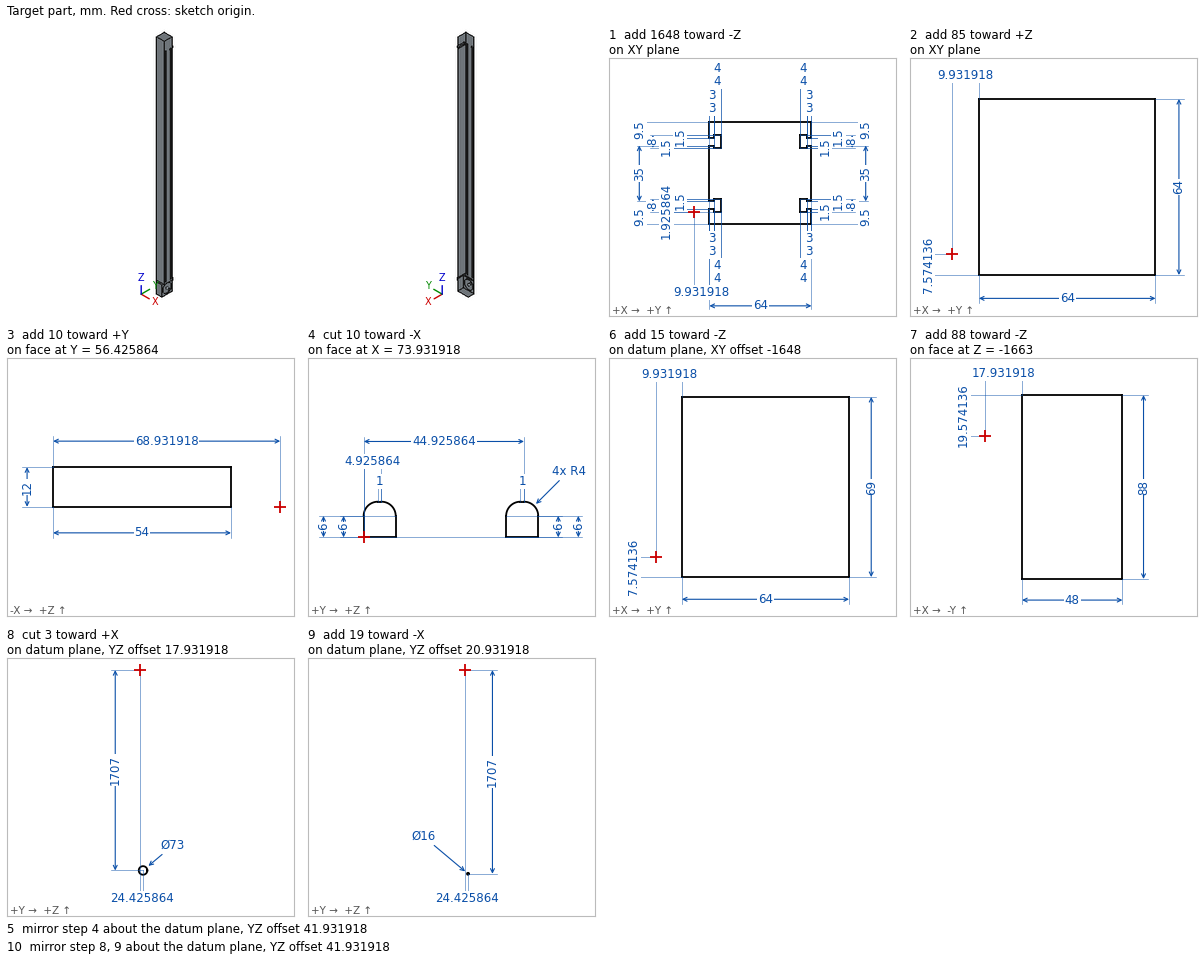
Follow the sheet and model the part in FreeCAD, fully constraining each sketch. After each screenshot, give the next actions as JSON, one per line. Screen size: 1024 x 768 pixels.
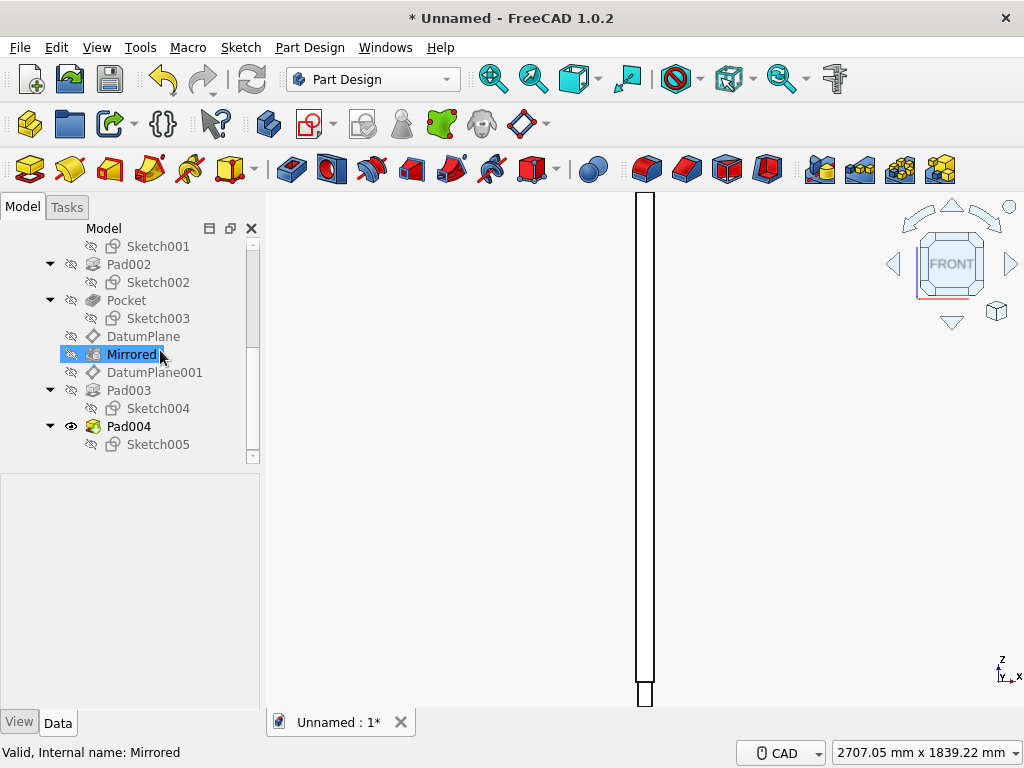
{"action": "scroll", "coordinate": [160, 350], "scroll_direction": "up", "scroll_amount": 15}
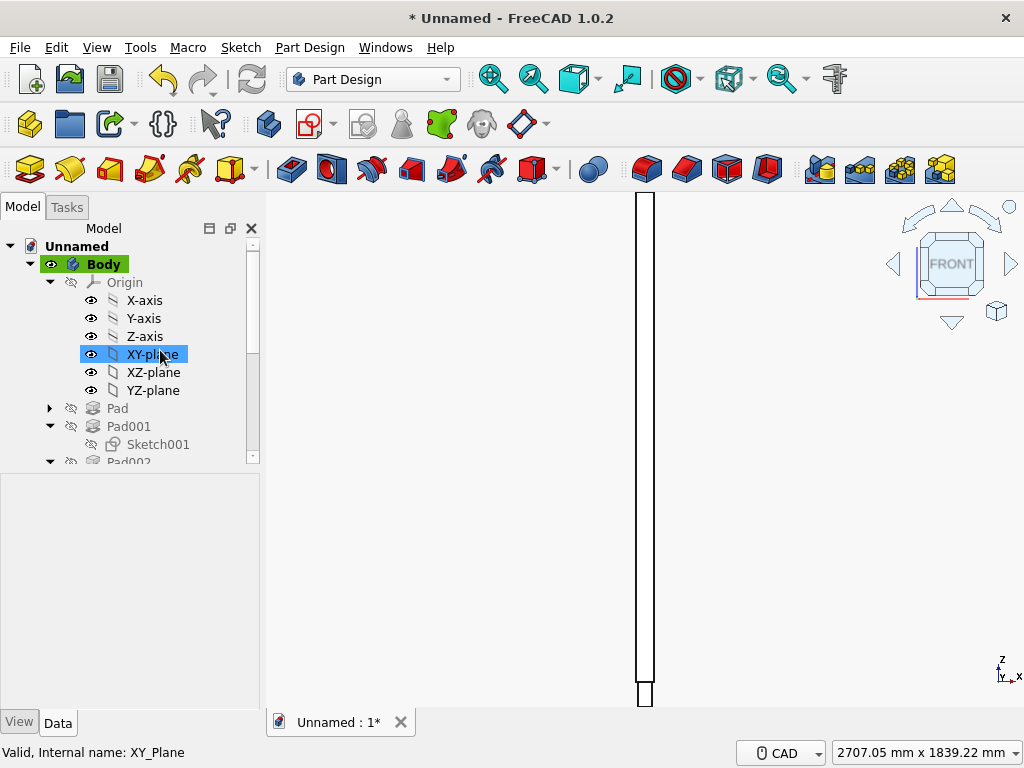
{"action": "left_click", "coordinate": [136, 390]}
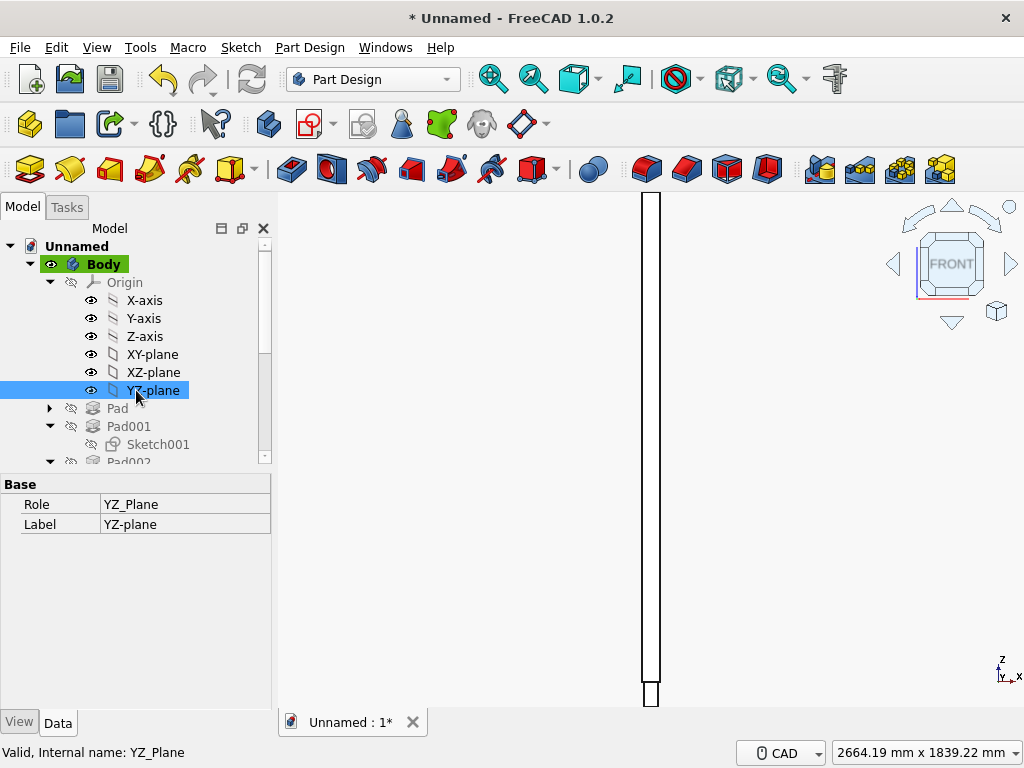
{"action": "left_click", "coordinate": [522, 124]}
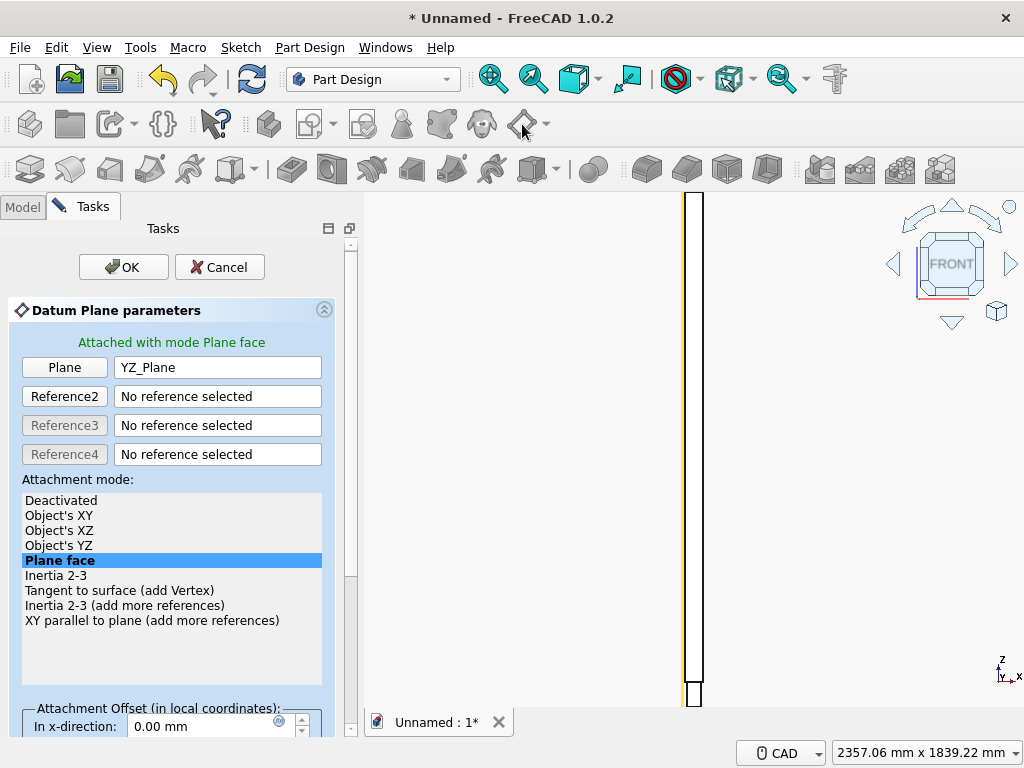
{"action": "scroll", "coordinate": [351, 487], "scroll_direction": "down", "scroll_amount": 3}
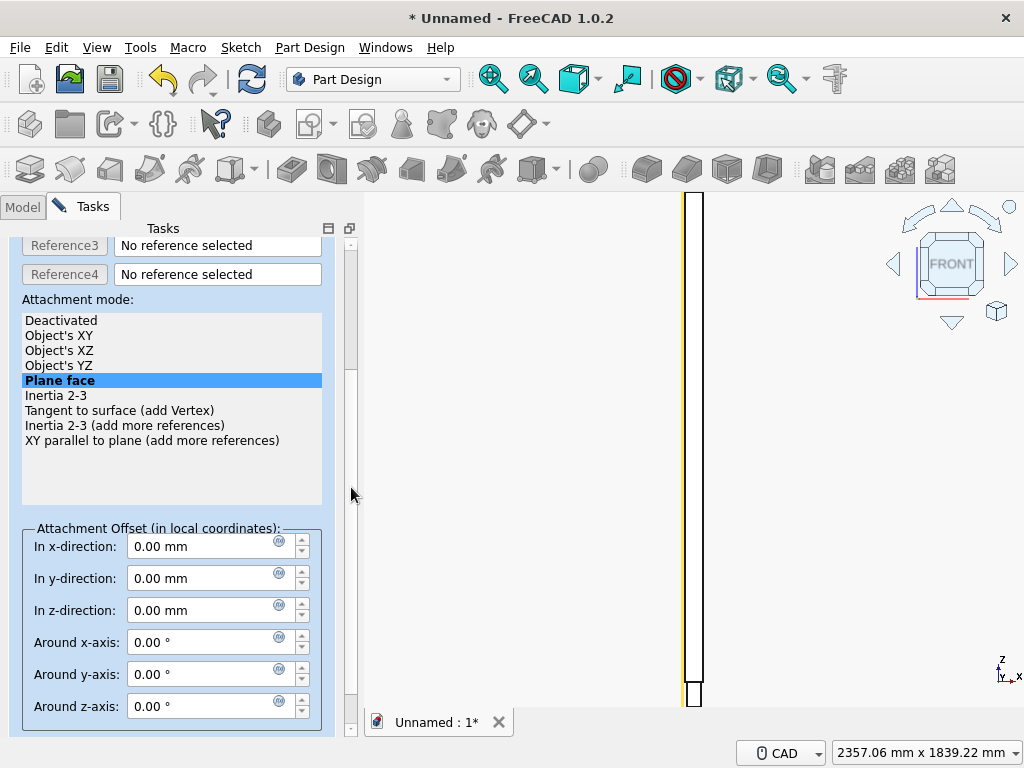
{"action": "triple_click", "coordinate": [210, 610]}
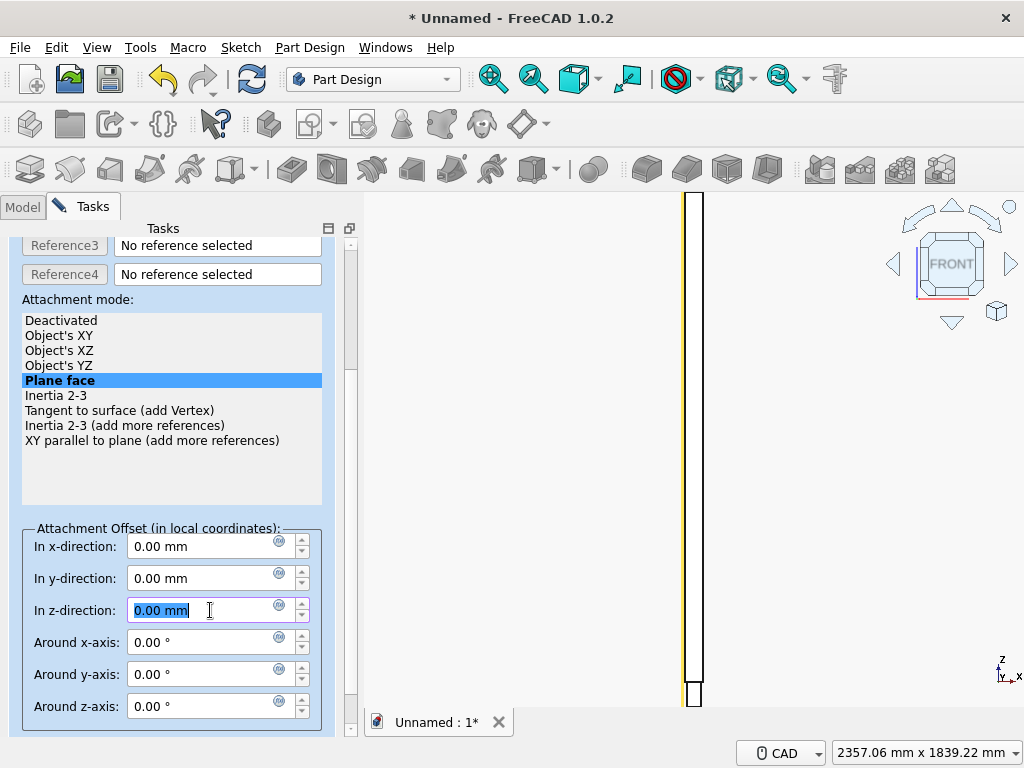
{"action": "type", "text": "17.931918"}
{"action": "key", "text": "Tab"}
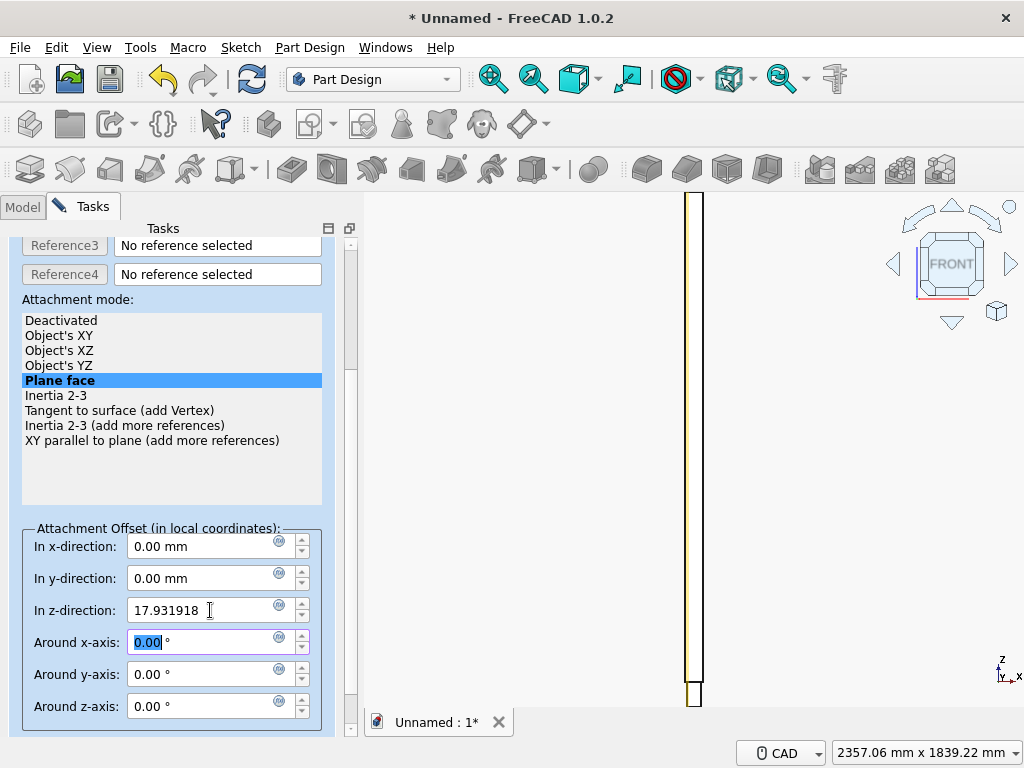
{"action": "scroll", "coordinate": [351, 487], "scroll_direction": "up", "scroll_amount": 4}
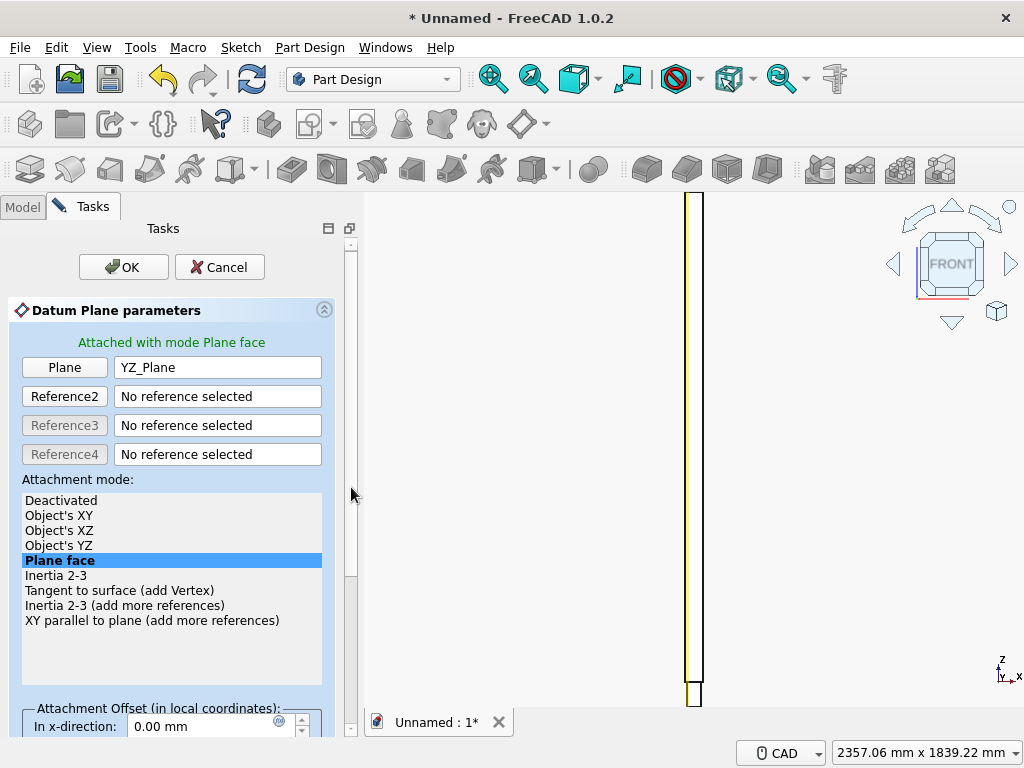
{"action": "left_click", "coordinate": [124, 267]}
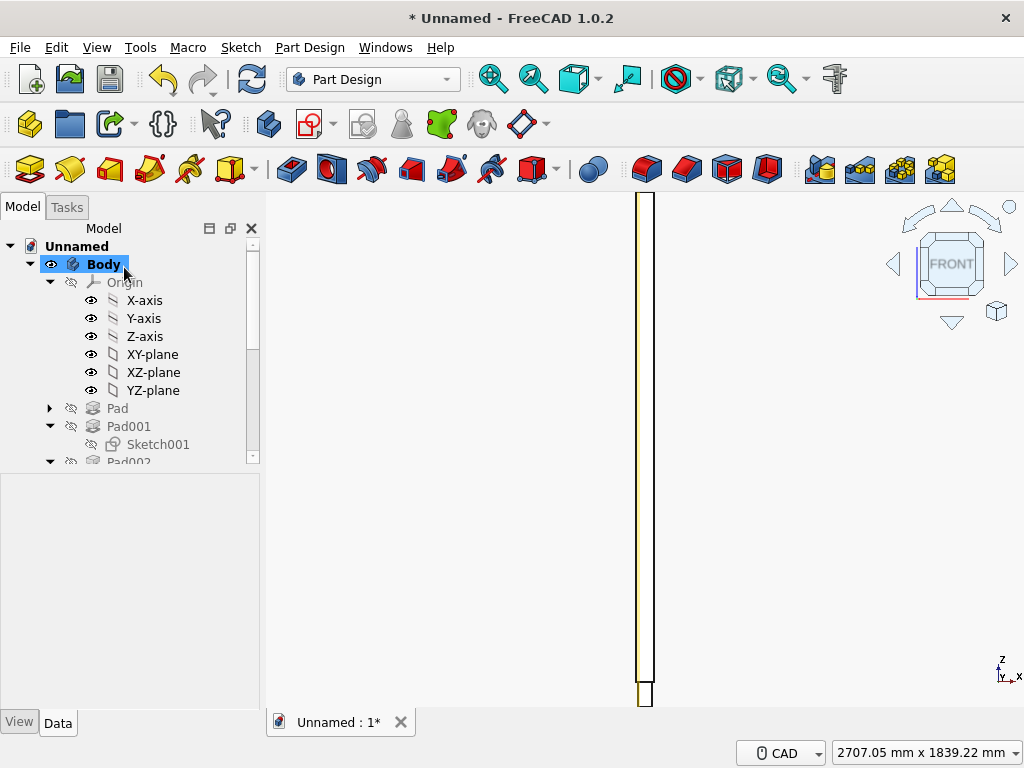
{"action": "scroll", "coordinate": [100, 350], "scroll_direction": "down", "scroll_amount": 3}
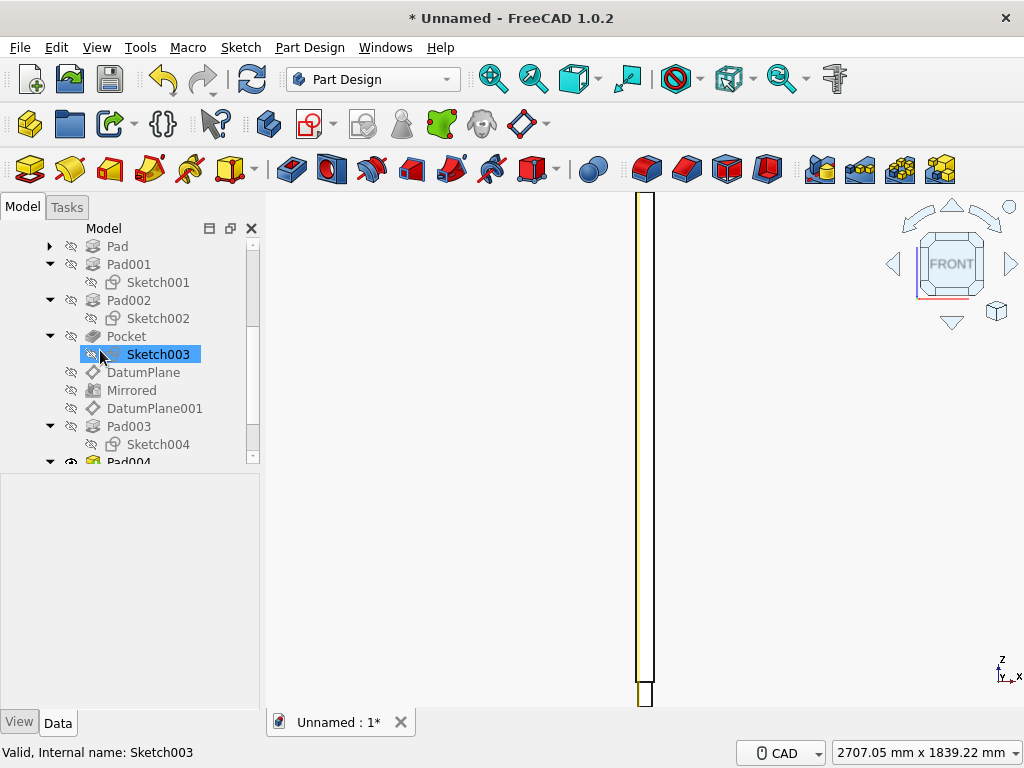
{"action": "scroll", "coordinate": [140, 350], "scroll_direction": "up", "scroll_amount": 15}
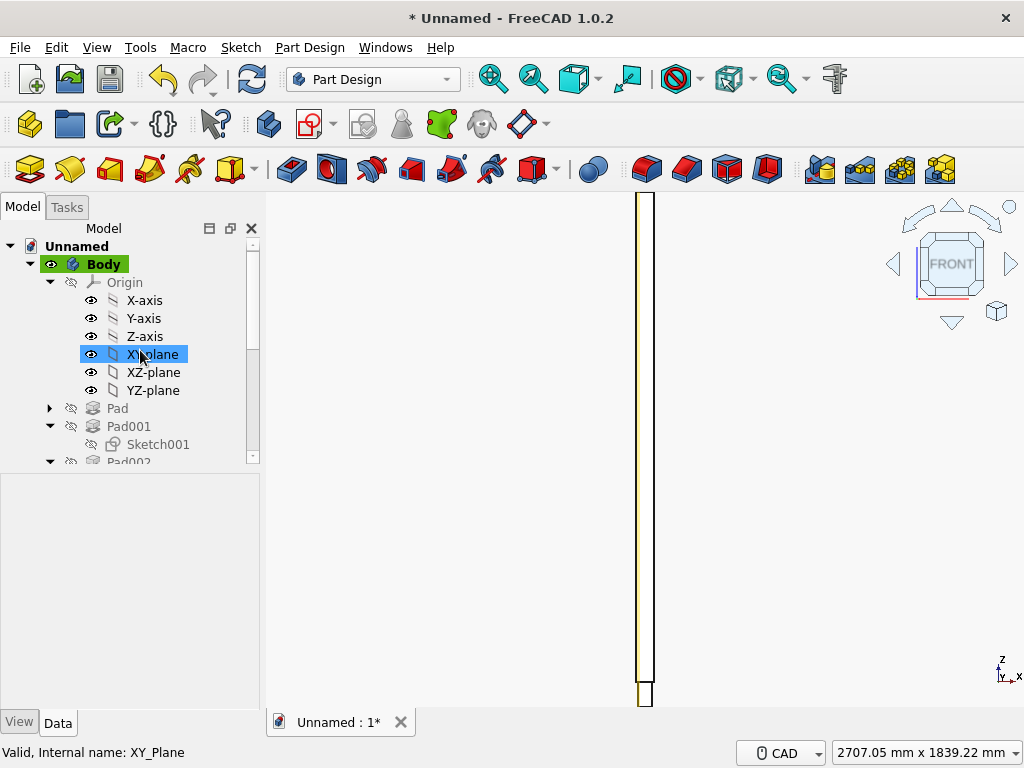
{"action": "scroll", "coordinate": [100, 350], "scroll_direction": "down", "scroll_amount": 6}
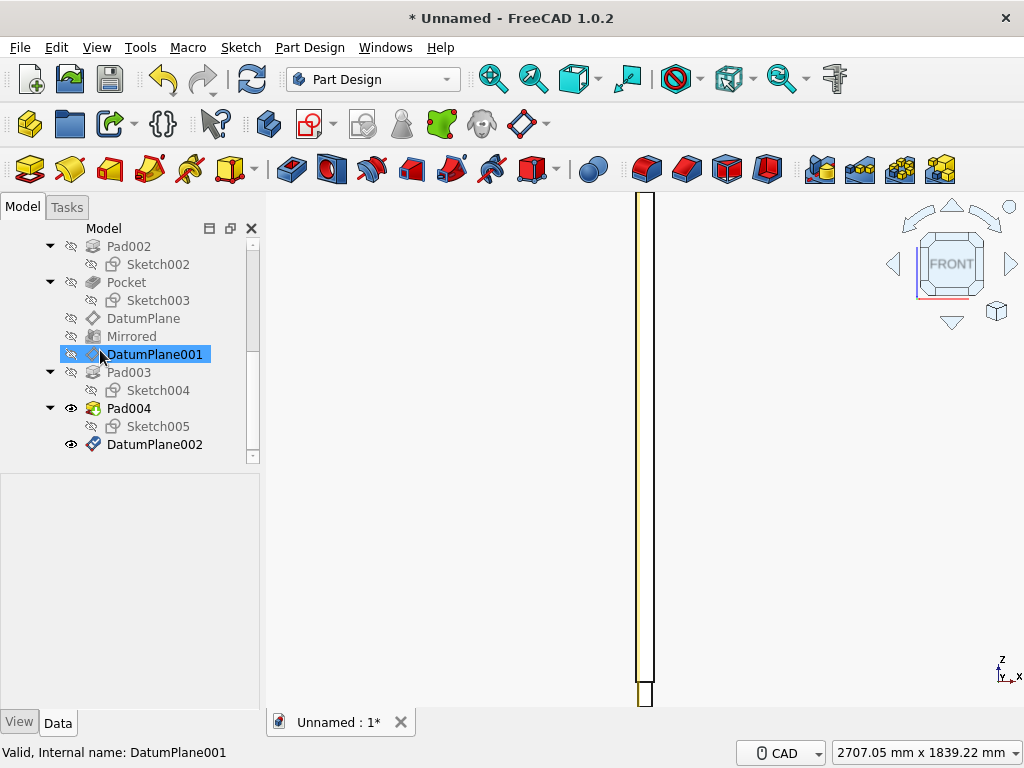
{"action": "left_click", "coordinate": [116, 444]}